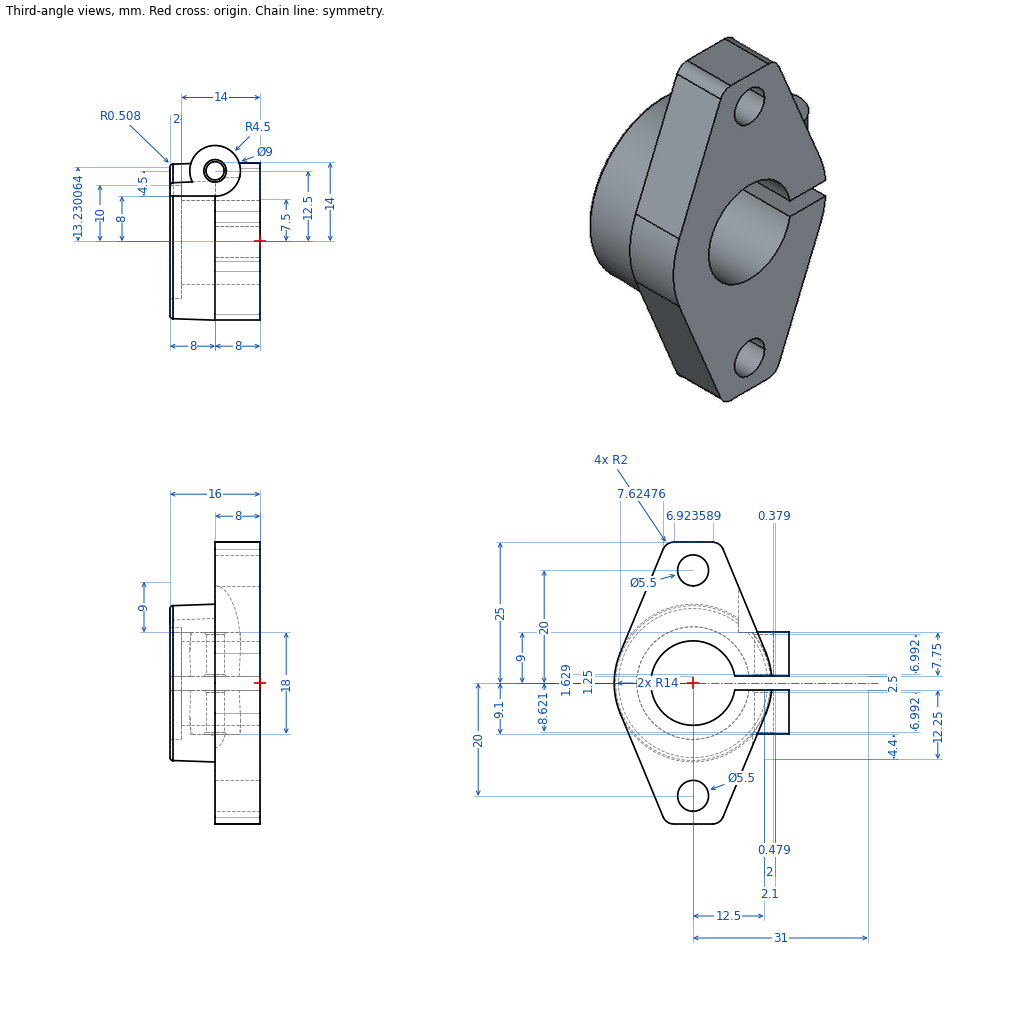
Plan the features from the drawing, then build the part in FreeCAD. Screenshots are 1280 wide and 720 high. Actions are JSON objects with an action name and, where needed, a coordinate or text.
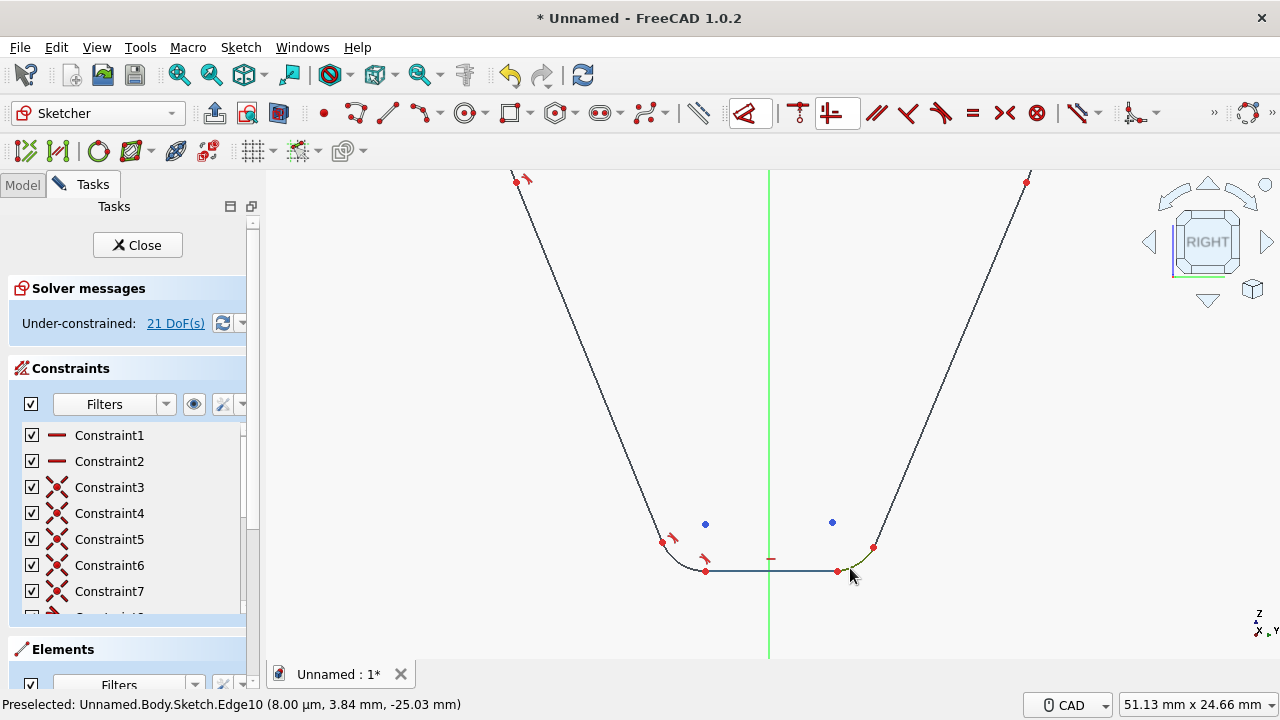
{"action": "left_click", "coordinate": [942, 114]}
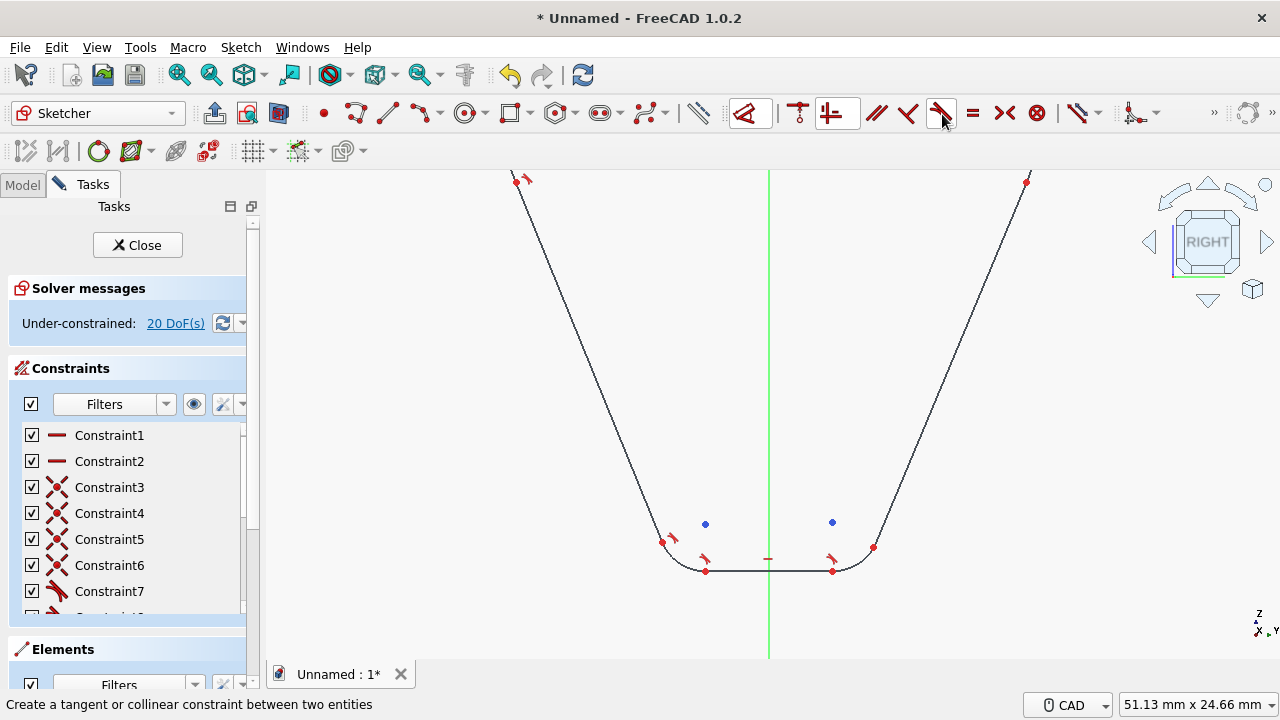
{"action": "scroll", "coordinate": [677, 562], "scroll_direction": "down", "scroll_amount": 6}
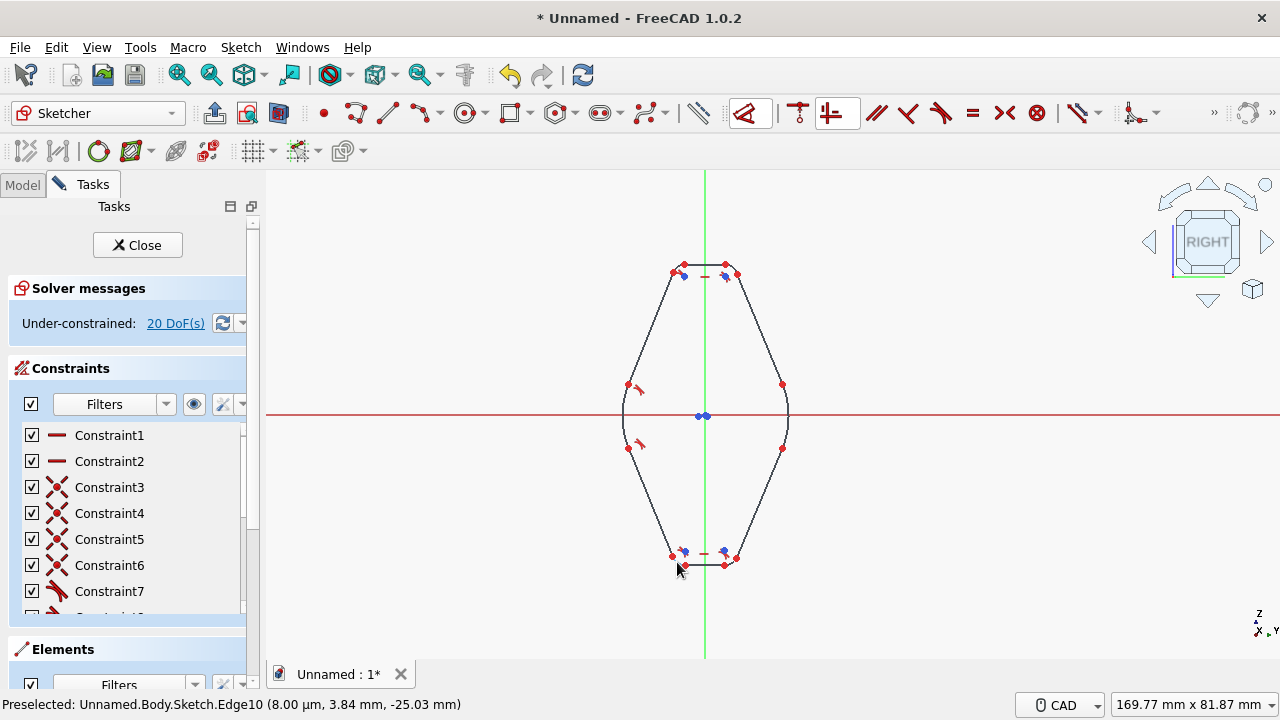
{"action": "left_click", "coordinate": [750, 525]}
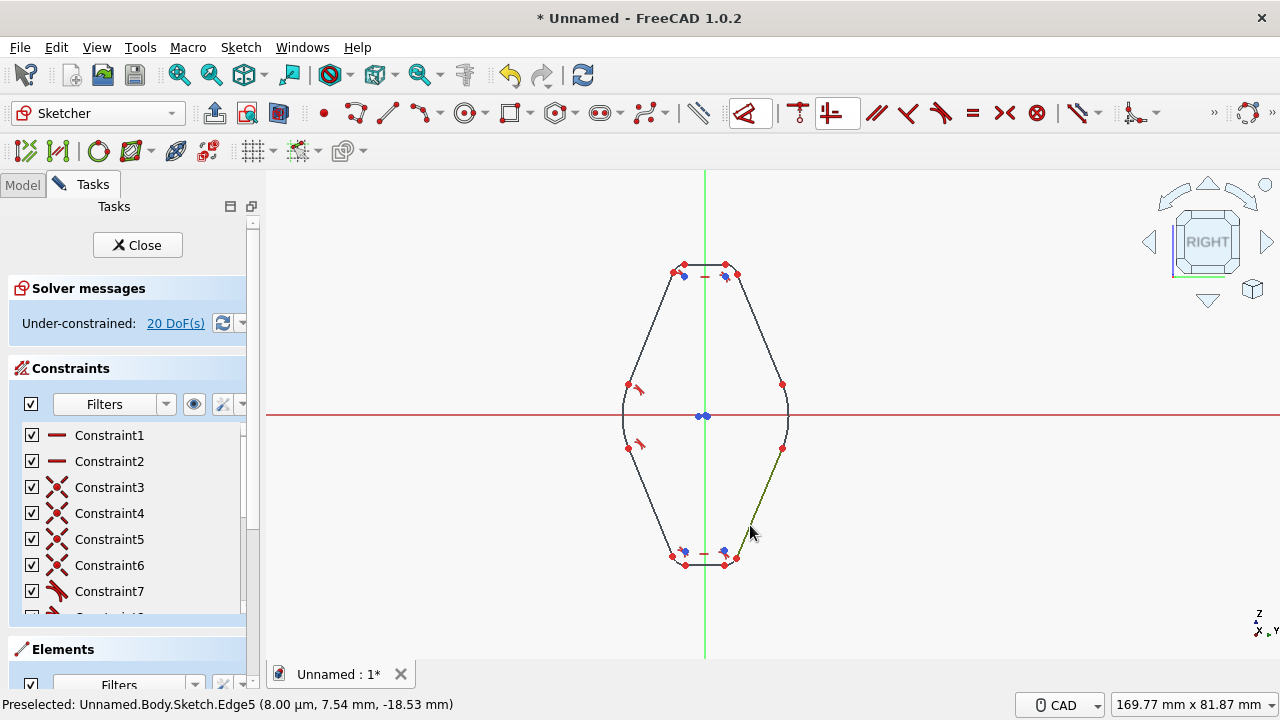
{"action": "scroll", "coordinate": [731, 563], "scroll_direction": "up", "scroll_amount": 4}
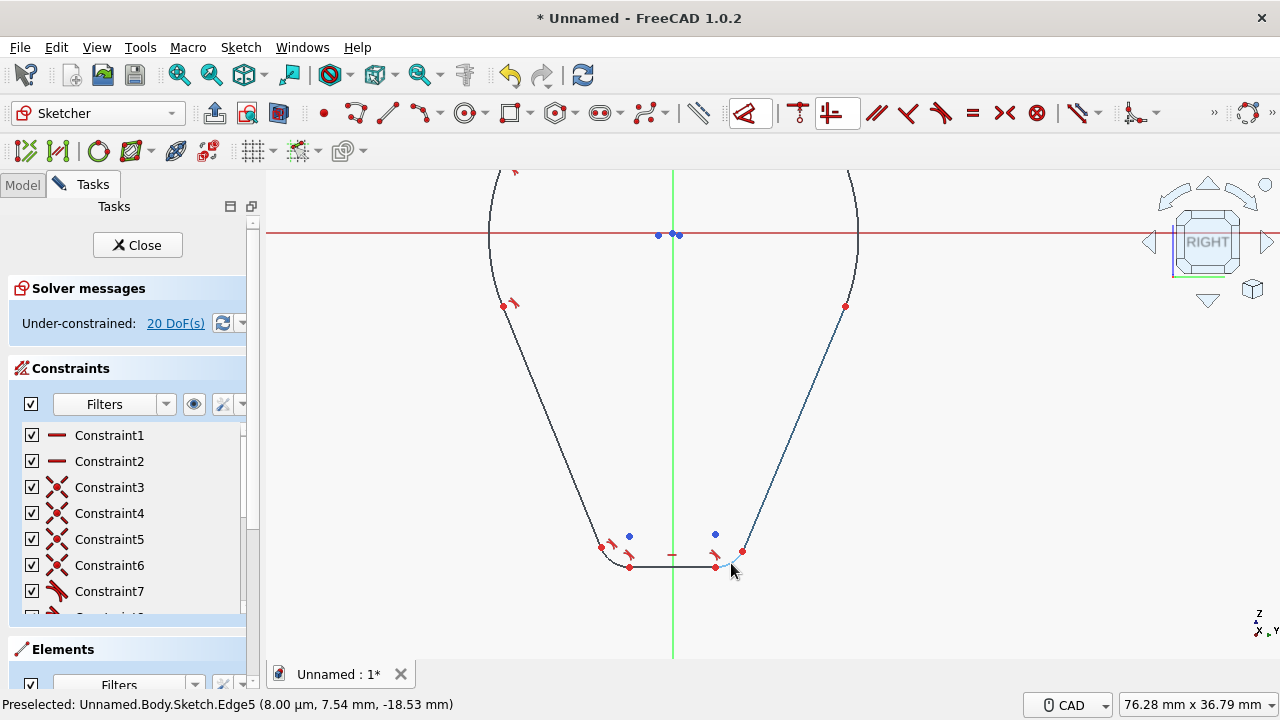
{"action": "left_click", "coordinate": [731, 563]}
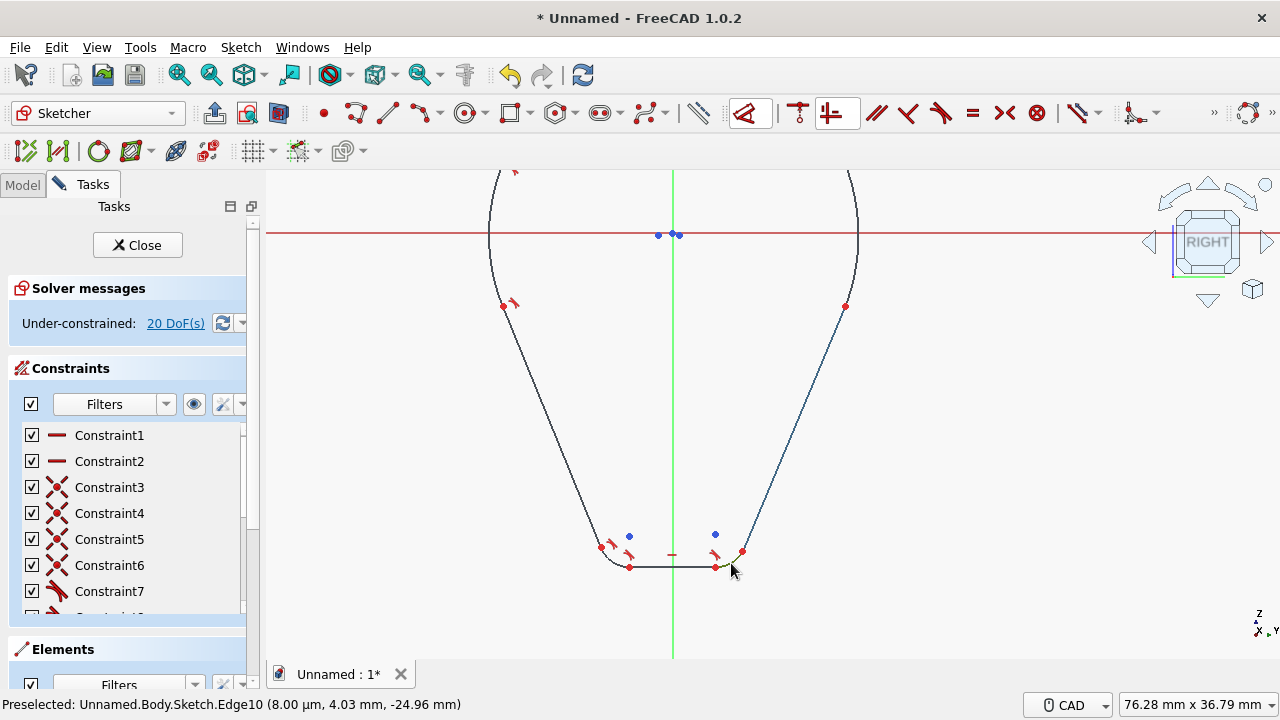
{"action": "key", "text": "t"}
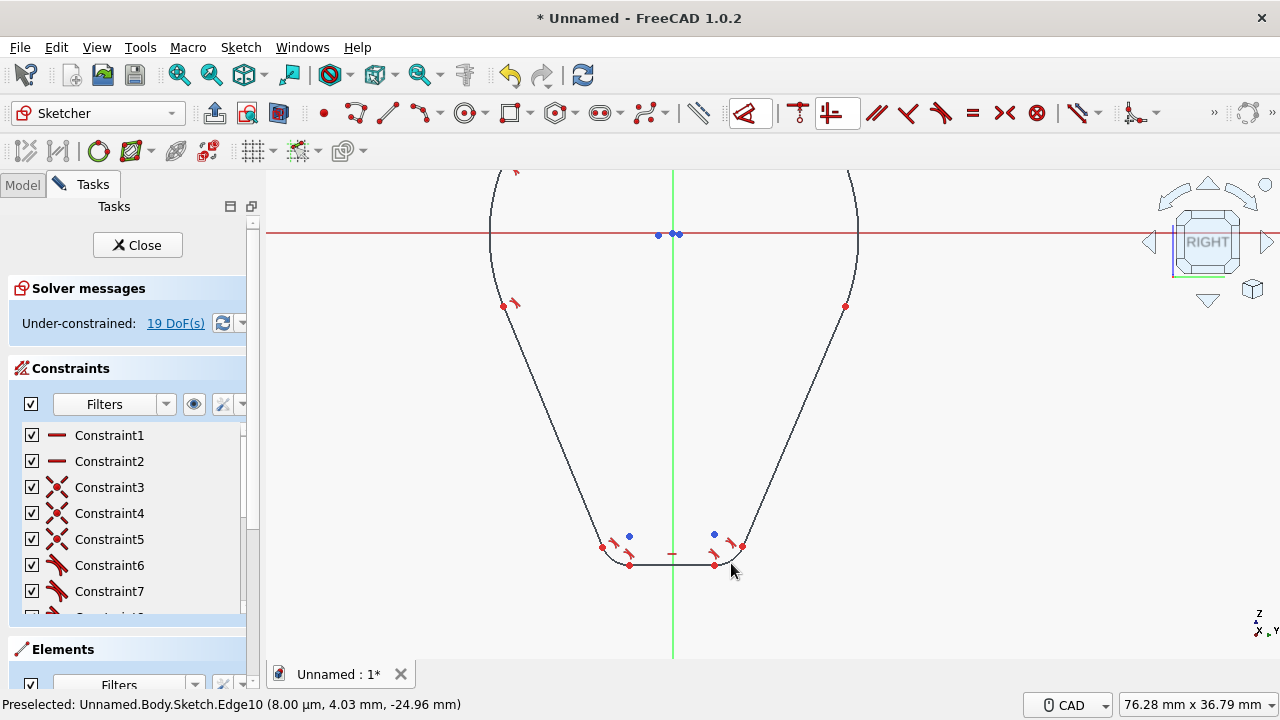
{"action": "left_click", "coordinate": [774, 475]}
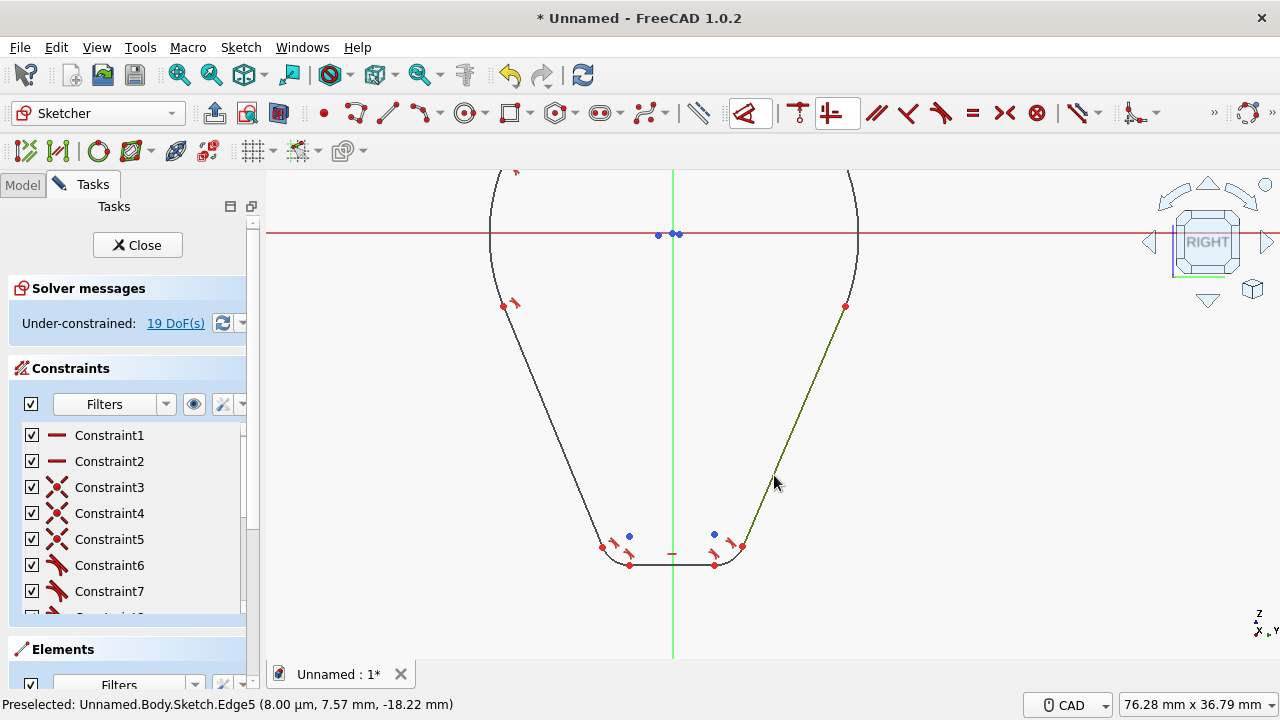
{"action": "left_click", "coordinate": [856, 265]}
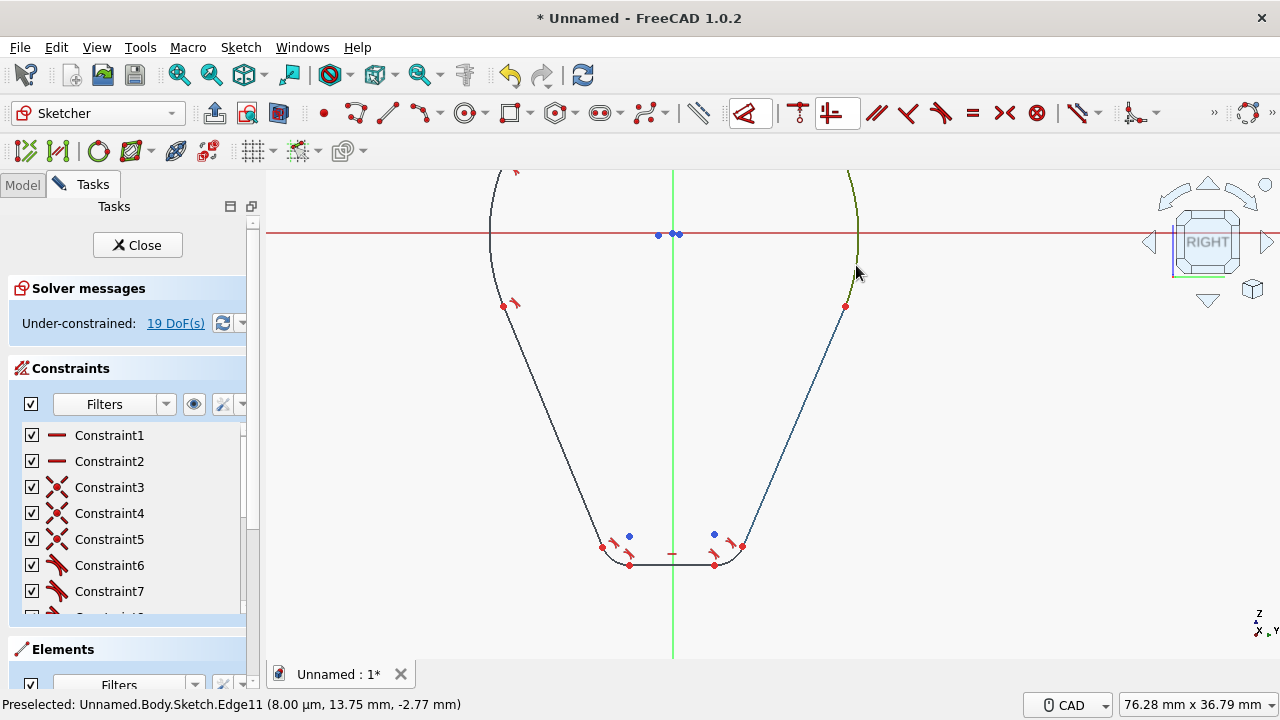
{"action": "key", "text": "t"}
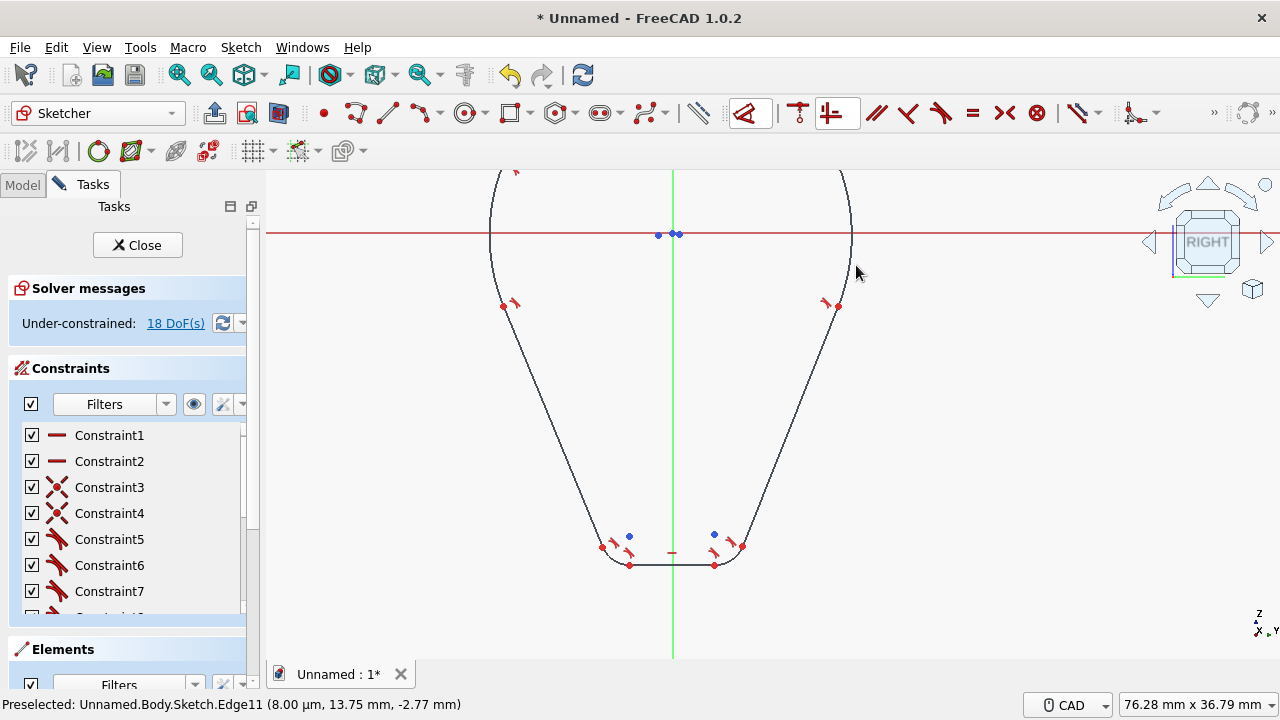
{"action": "scroll", "coordinate": [730, 562], "scroll_direction": "down", "scroll_amount": 4}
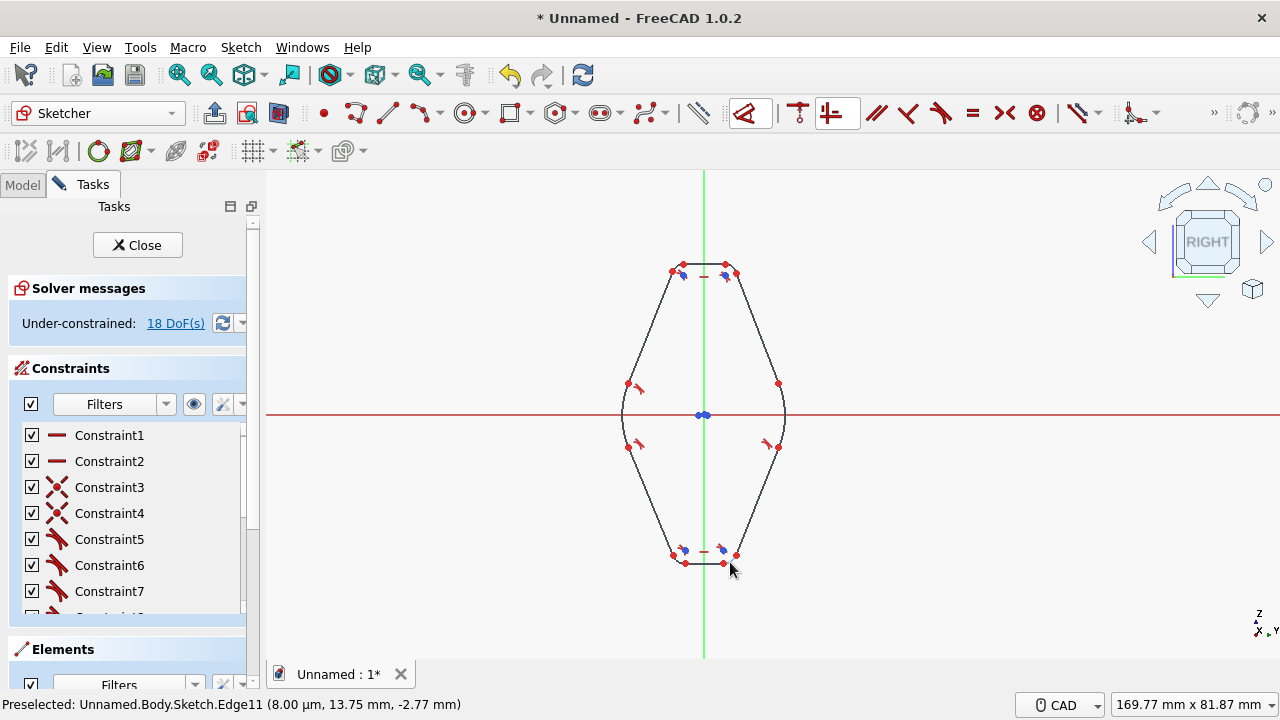
{"action": "left_click", "coordinate": [766, 351]}